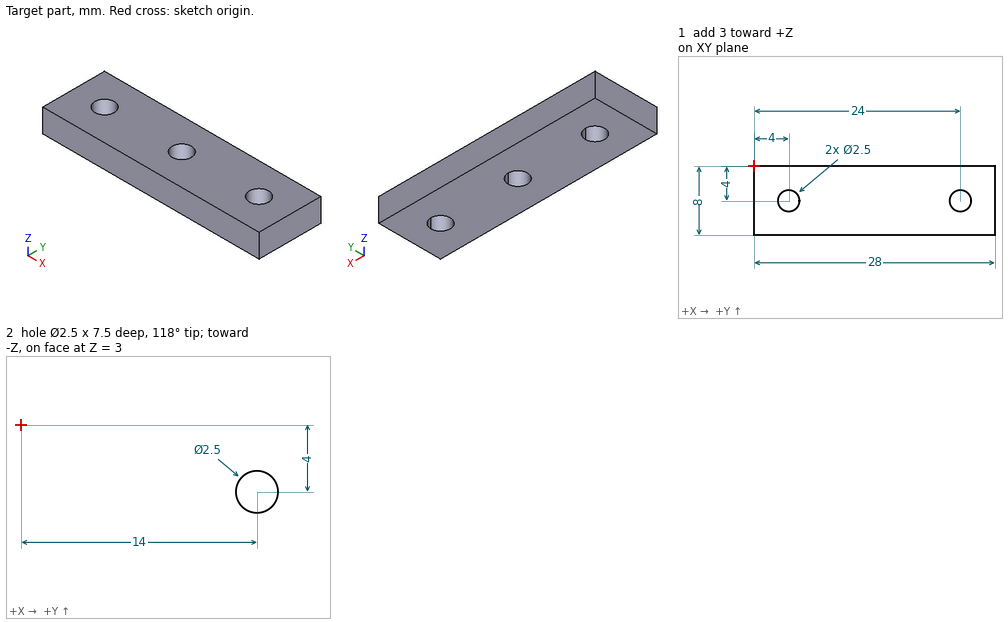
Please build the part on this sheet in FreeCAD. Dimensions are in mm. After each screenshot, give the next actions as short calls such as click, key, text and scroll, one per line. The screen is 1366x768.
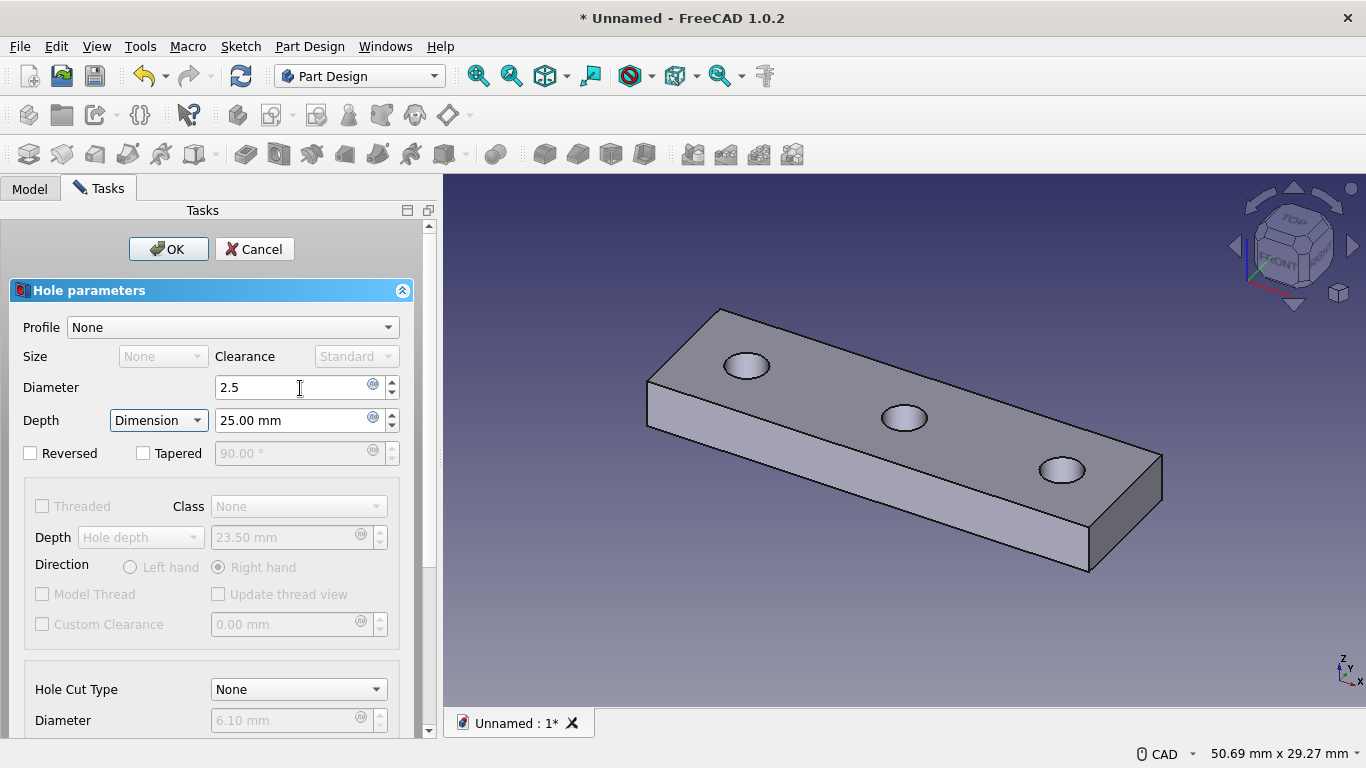
triple_click(300, 420)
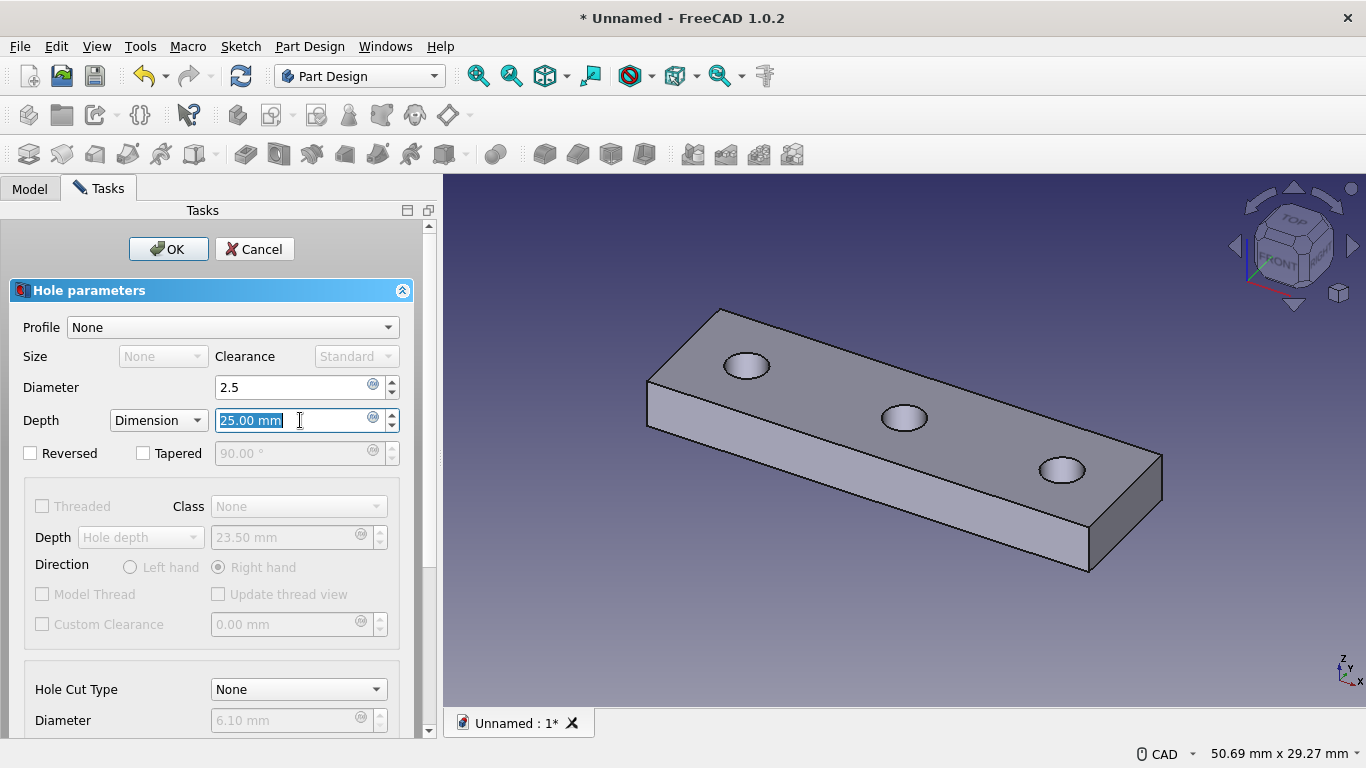
text(7.5)
key(Tab)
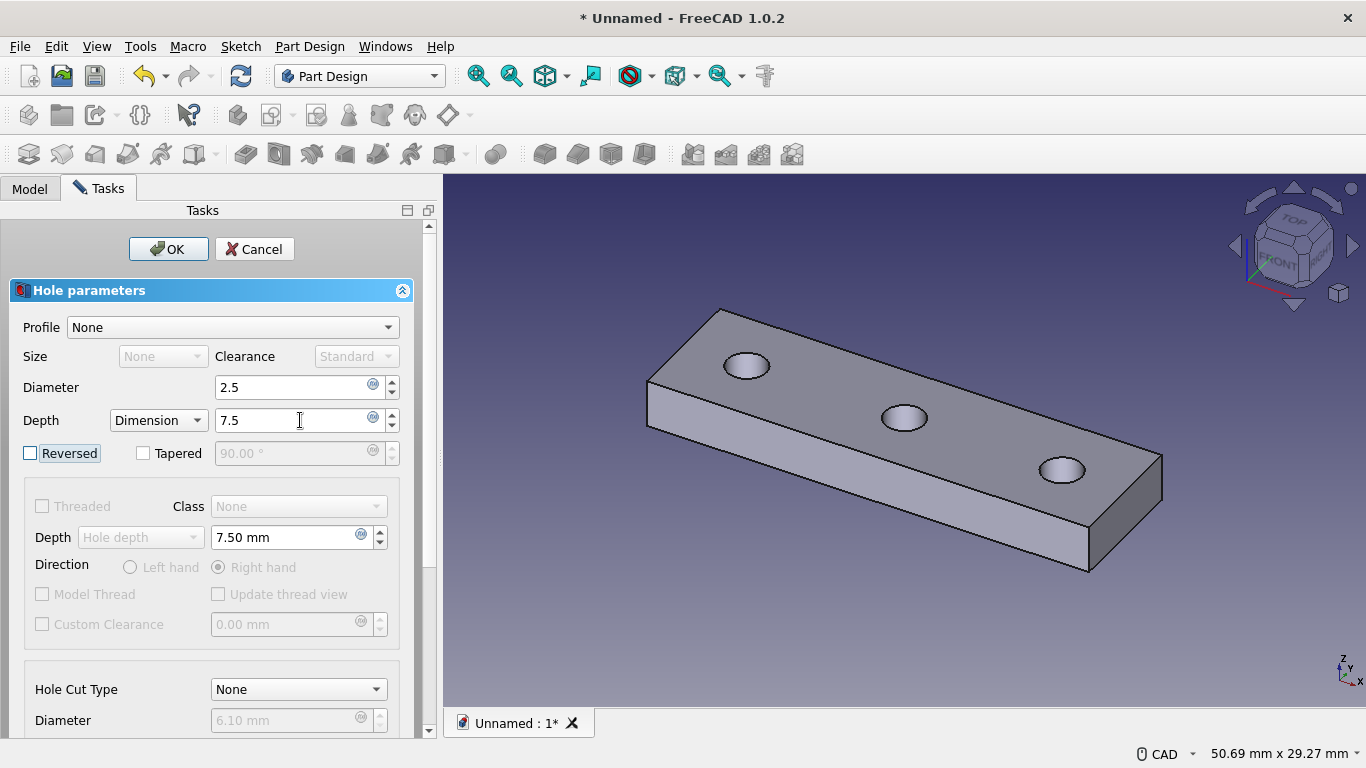
click(169, 249)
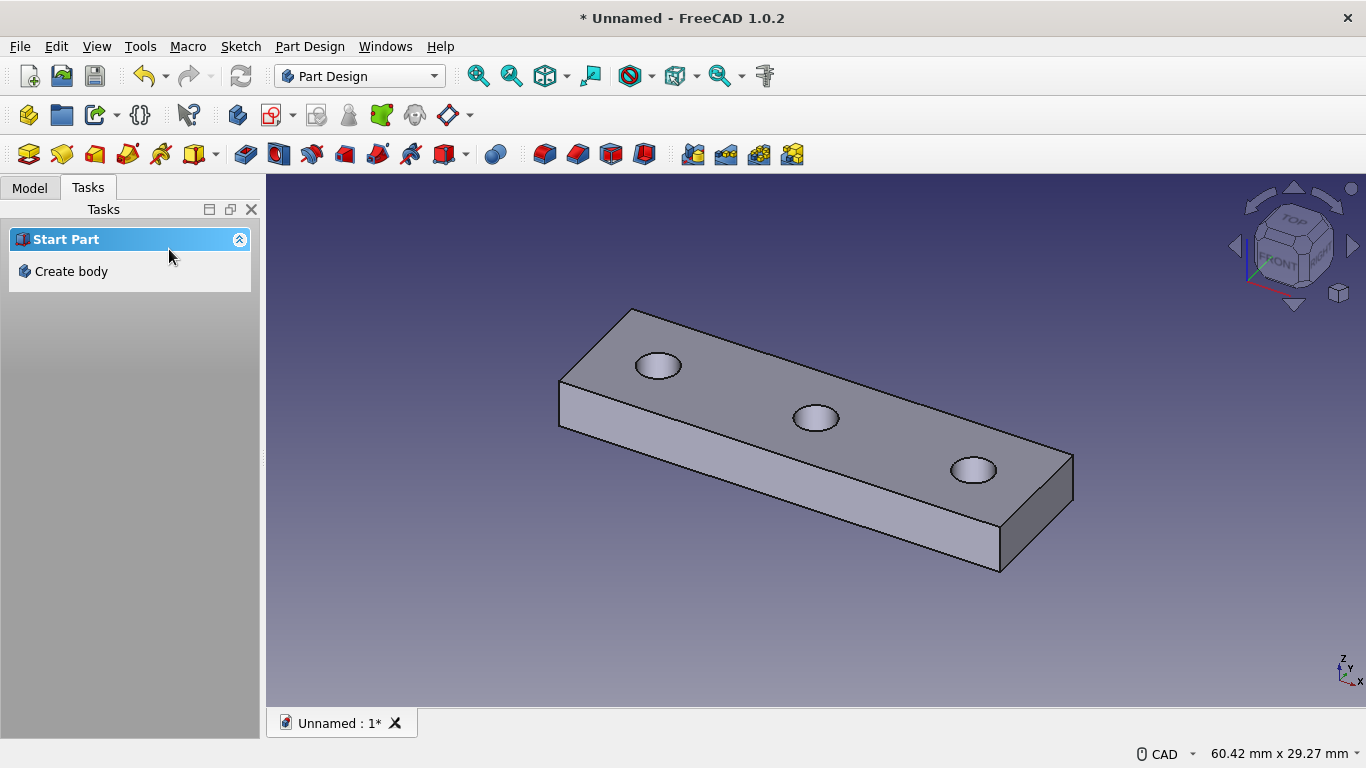
key(0)